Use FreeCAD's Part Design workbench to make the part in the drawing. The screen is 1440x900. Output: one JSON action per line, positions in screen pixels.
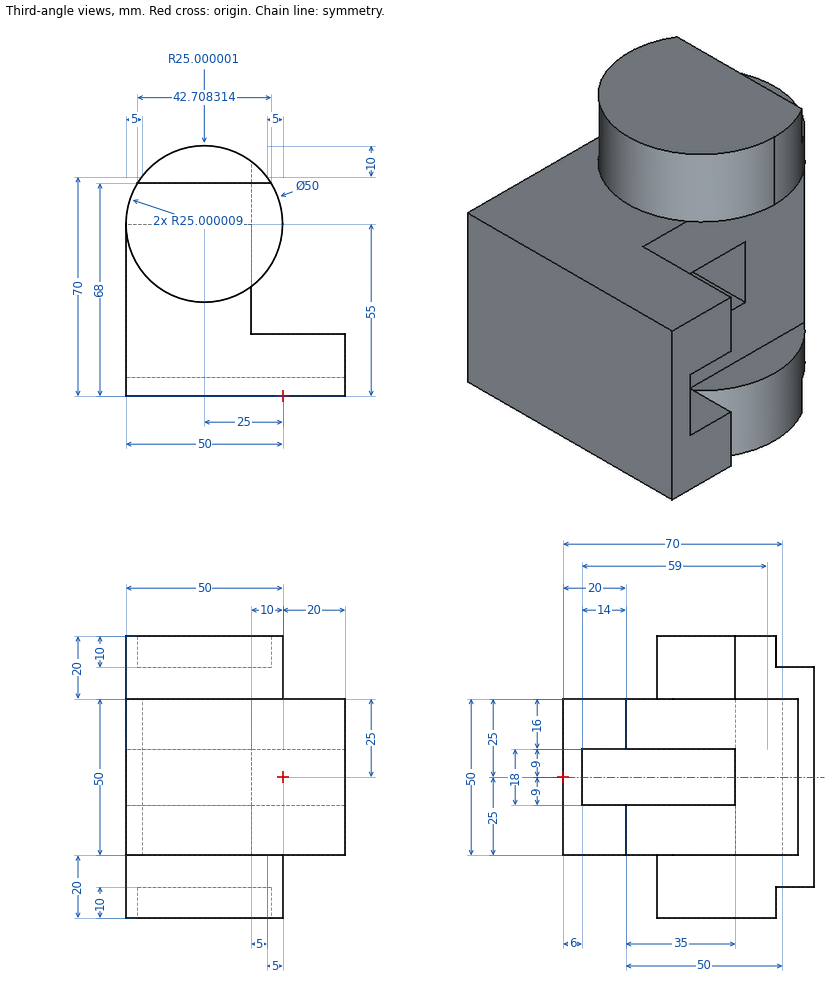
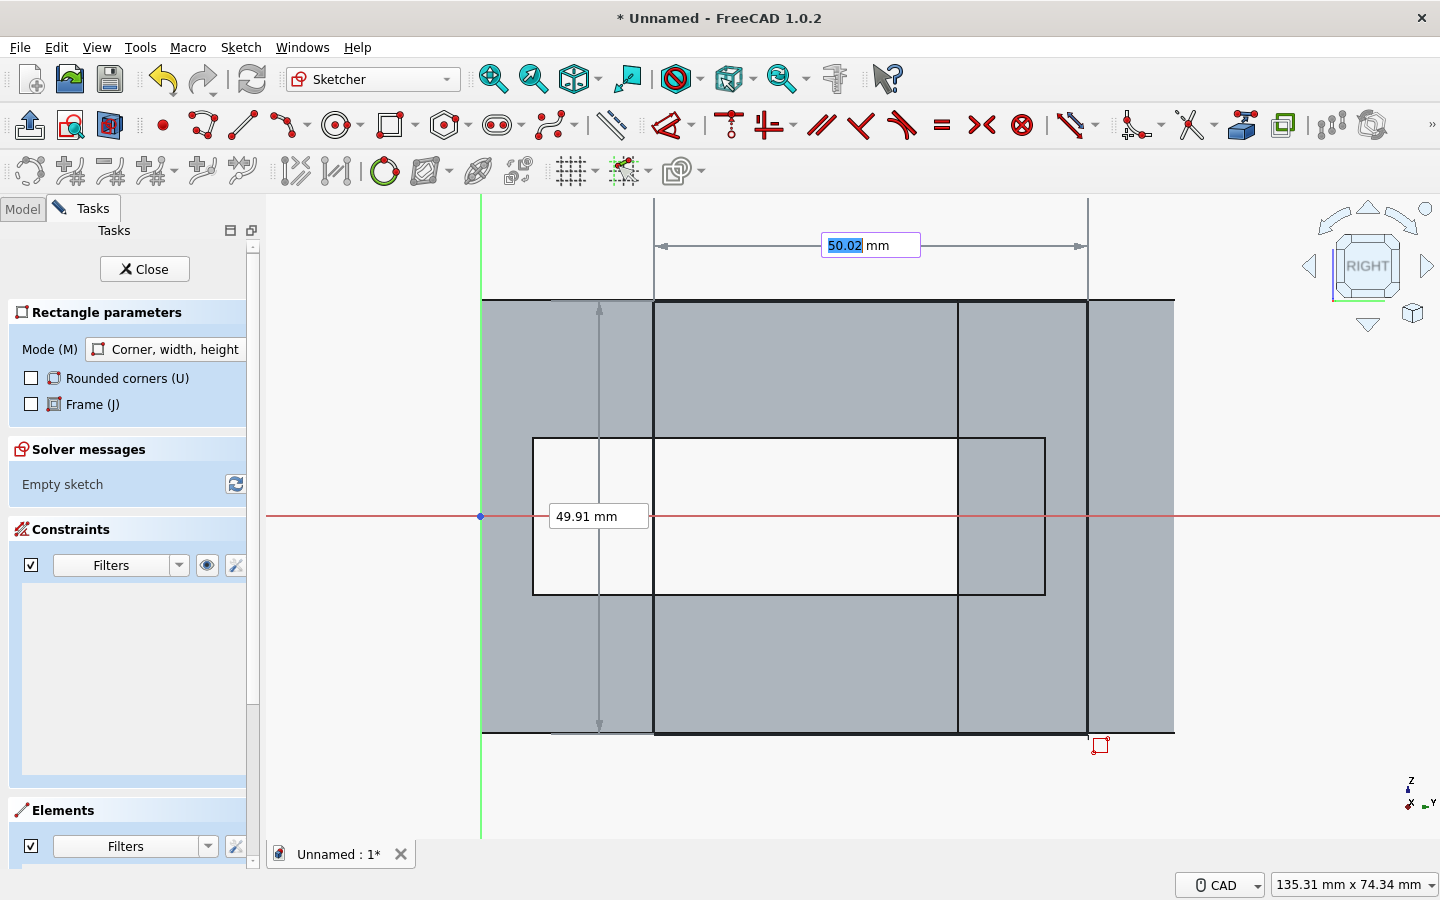
{"action": "type", "text": "50"}
{"action": "key", "text": "Tab"}
{"action": "type", "text": "50"}
{"action": "key", "text": "Return"}
{"action": "key", "text": "Escape"}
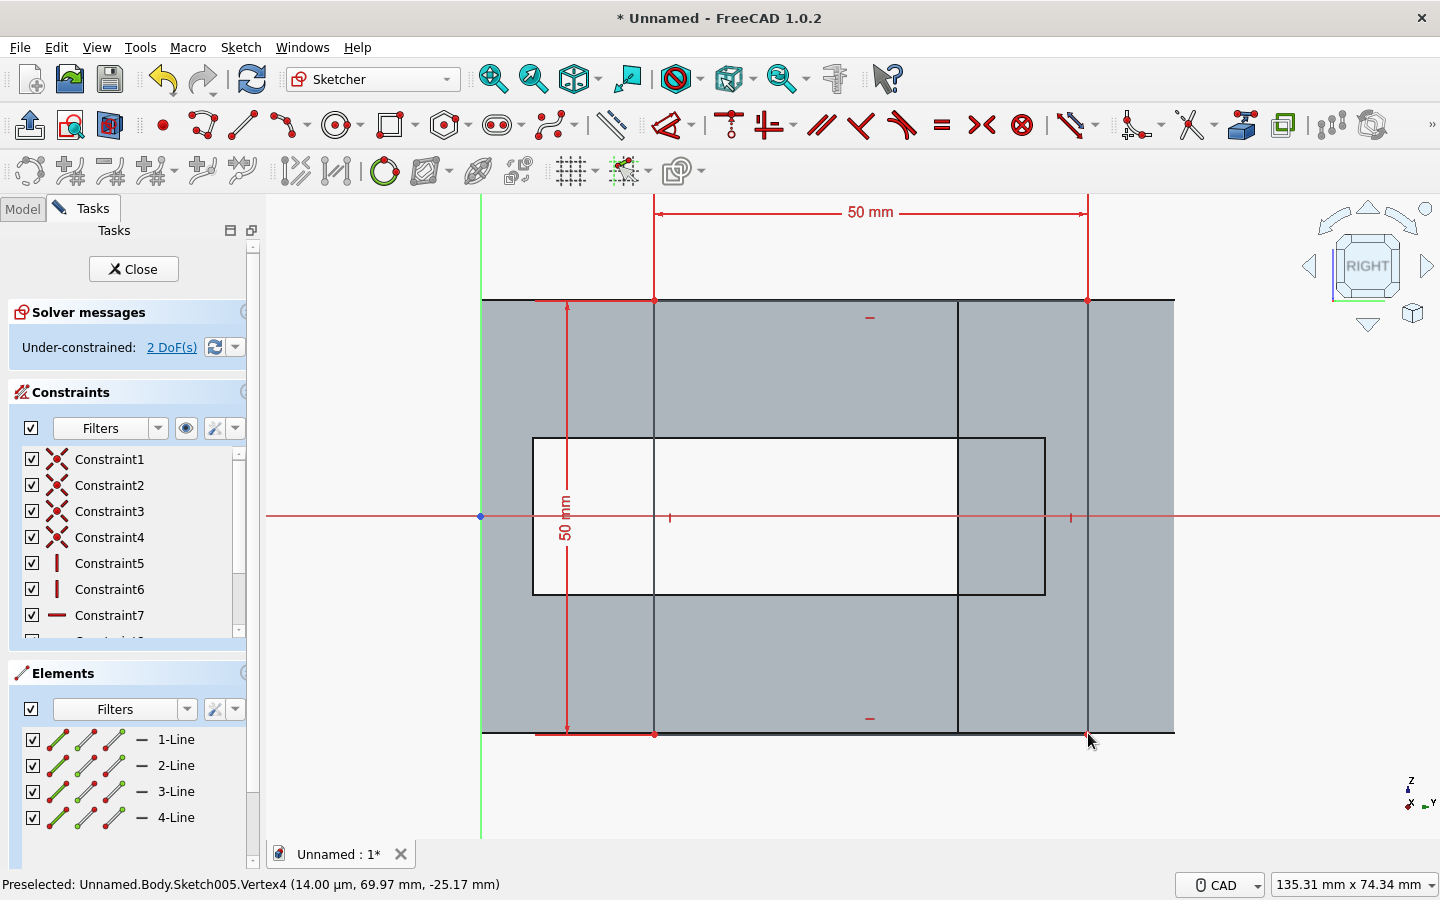
{"action": "key", "text": "d"}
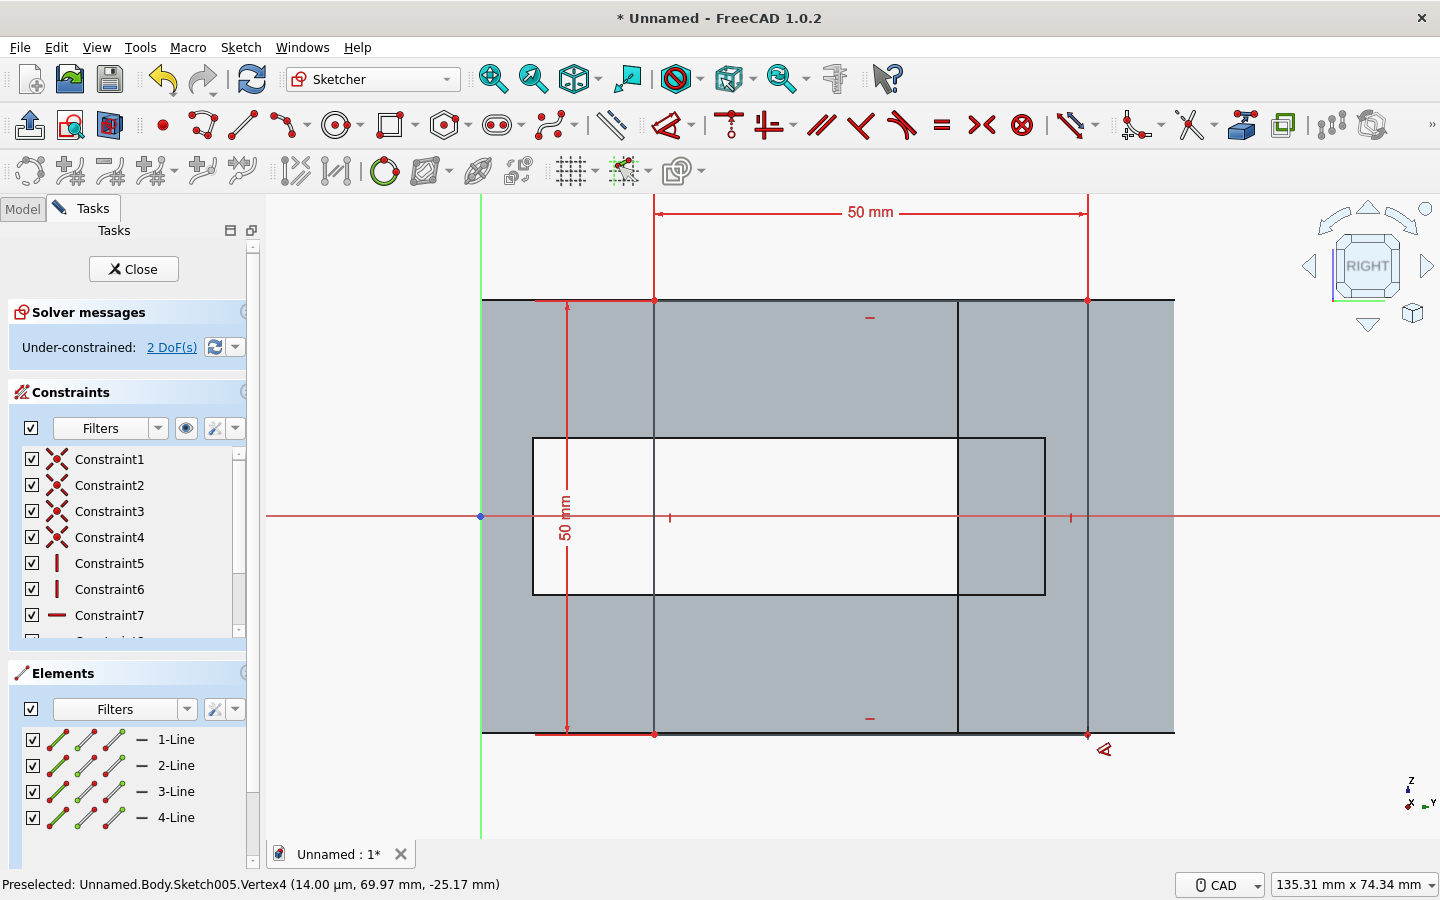
{"action": "left_click", "coordinate": [654, 301]}
{"action": "left_click", "coordinate": [567, 267]}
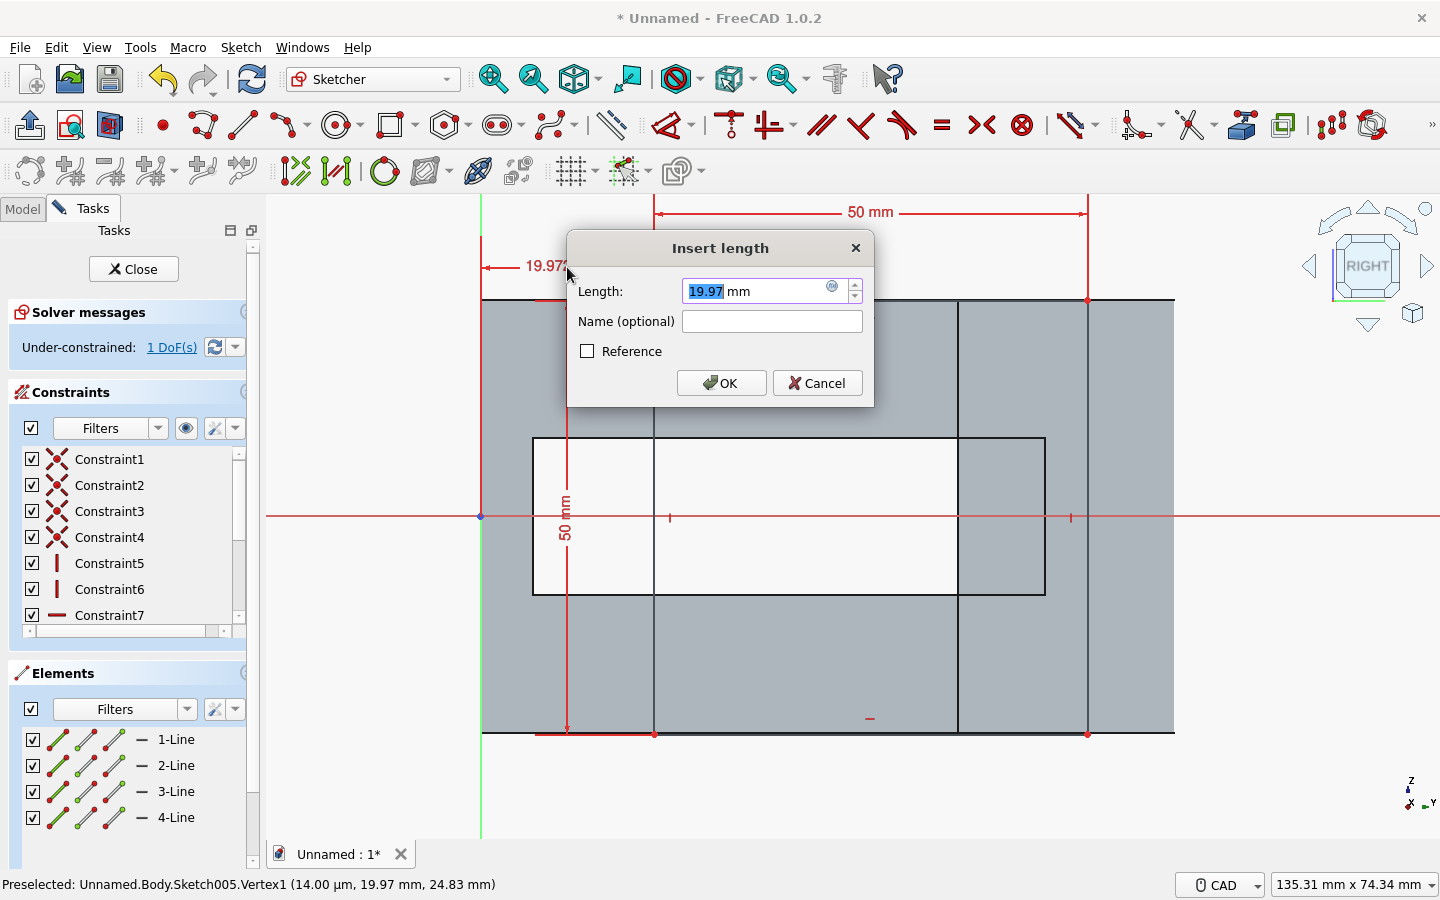
{"action": "type", "text": "20"}
{"action": "key", "text": "Return"}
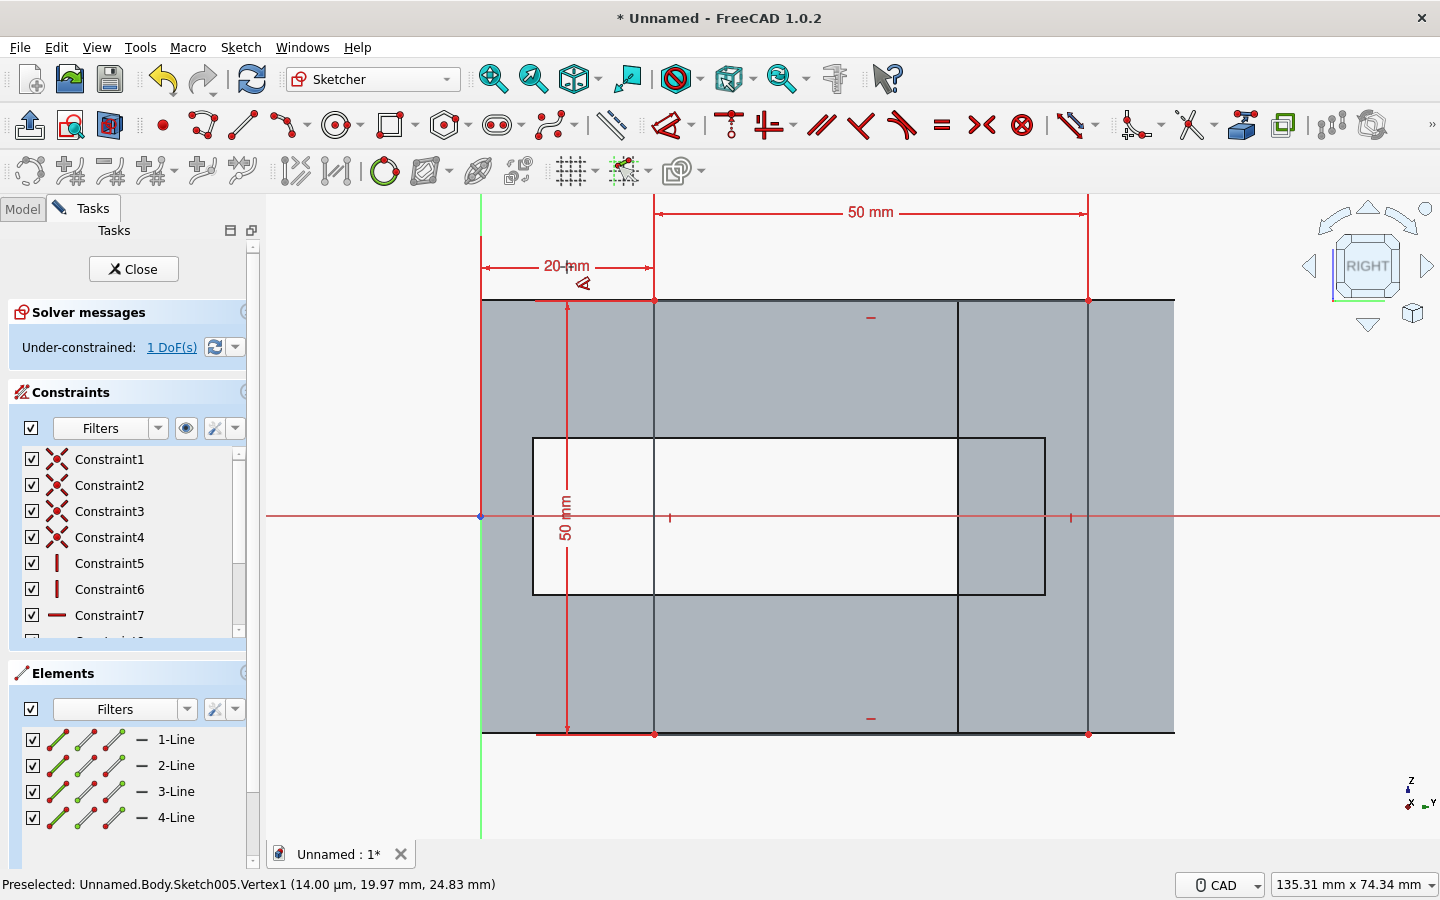
{"action": "left_click", "coordinate": [654, 301]}
{"action": "left_click", "coordinate": [447, 409]}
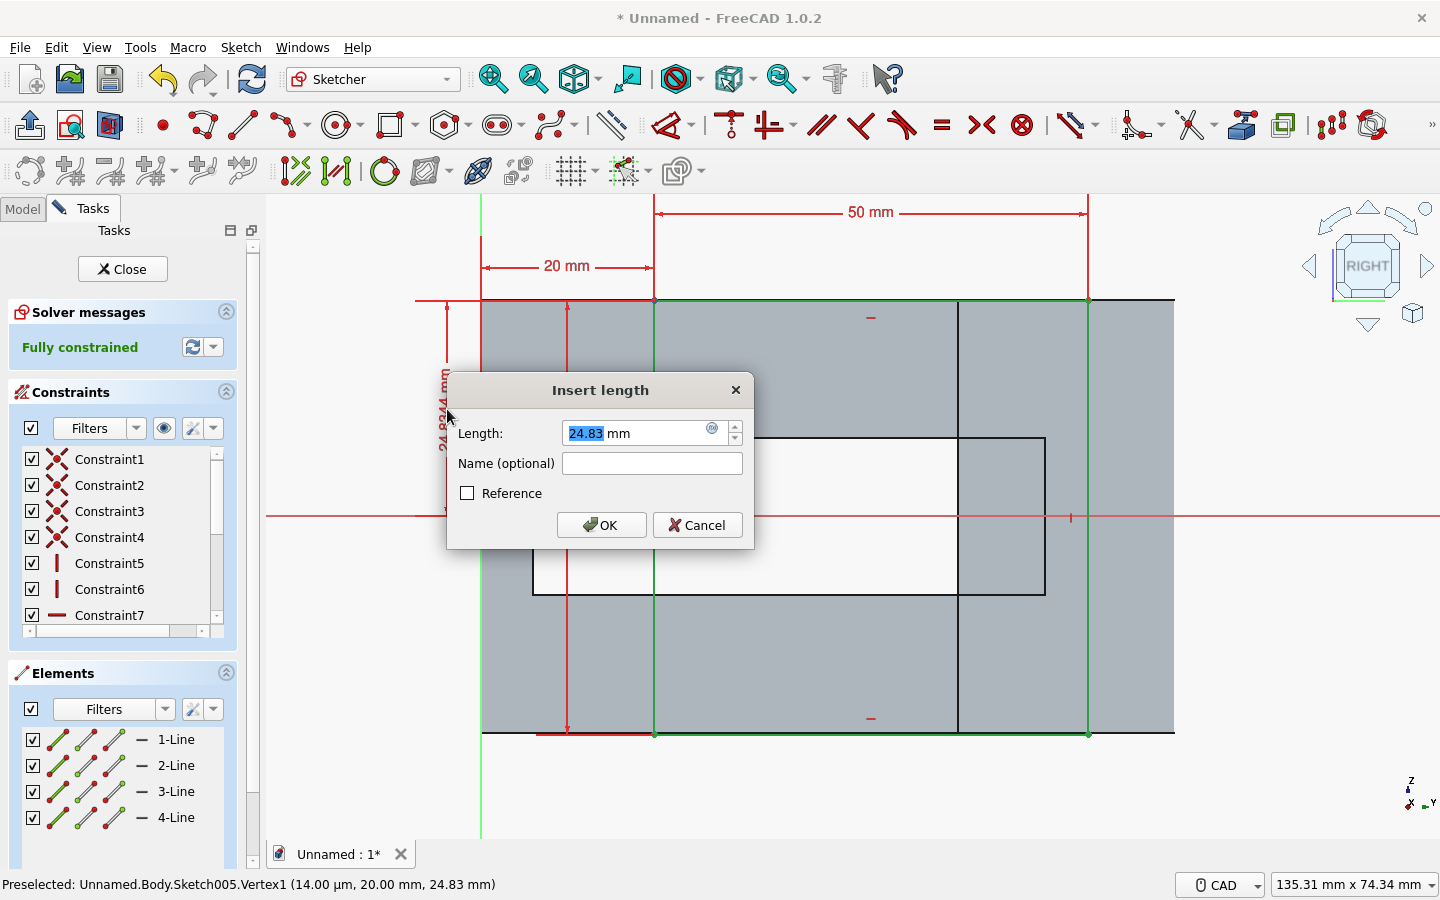
{"action": "type", "text": "25"}
{"action": "key", "text": "Return"}
{"action": "key", "text": "Escape"}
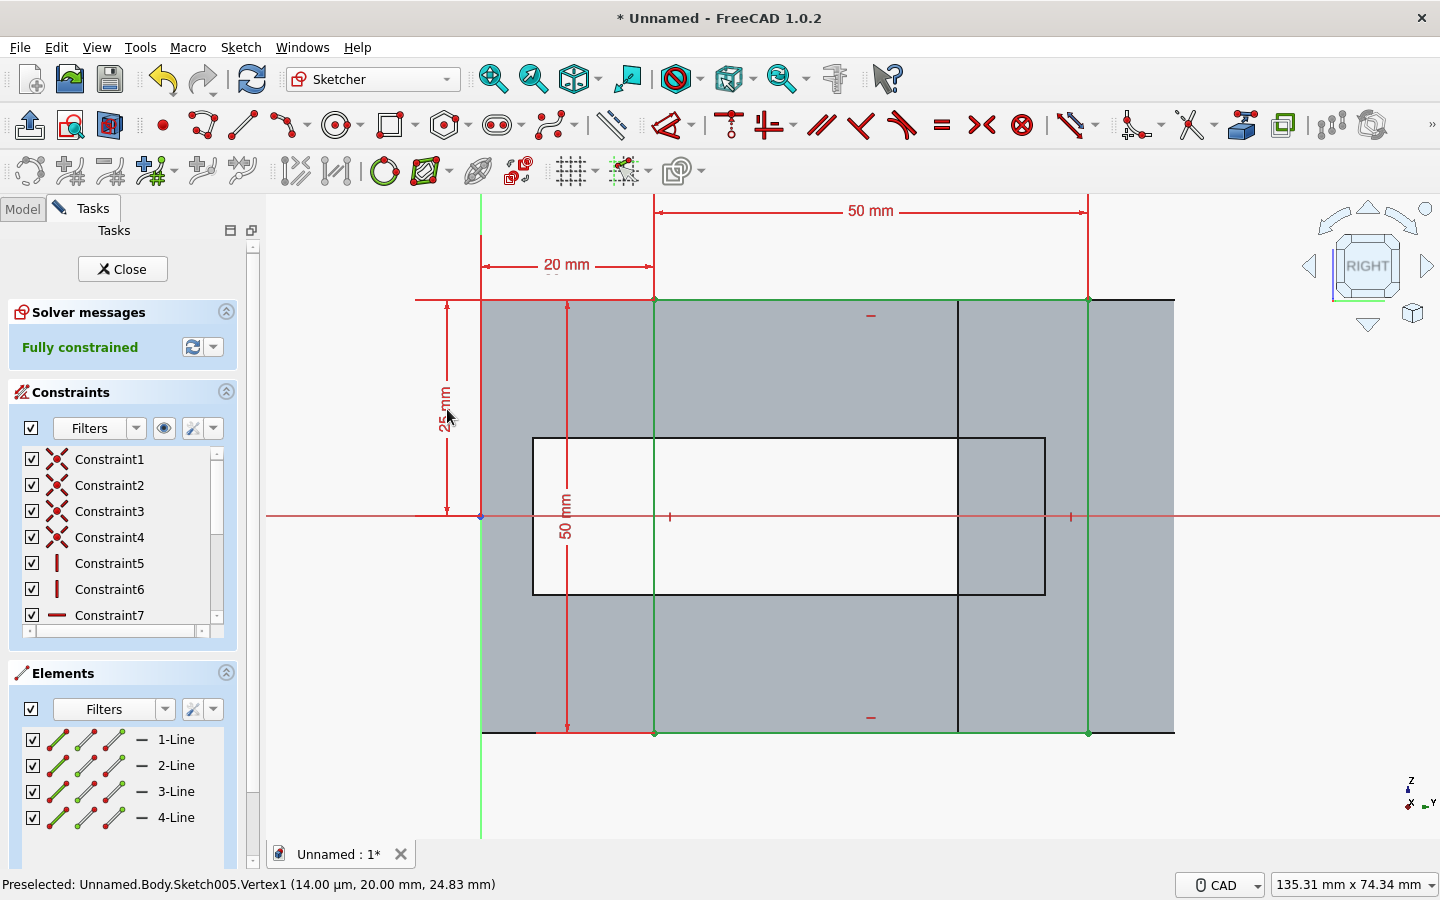
{"action": "left_click", "coordinate": [123, 269]}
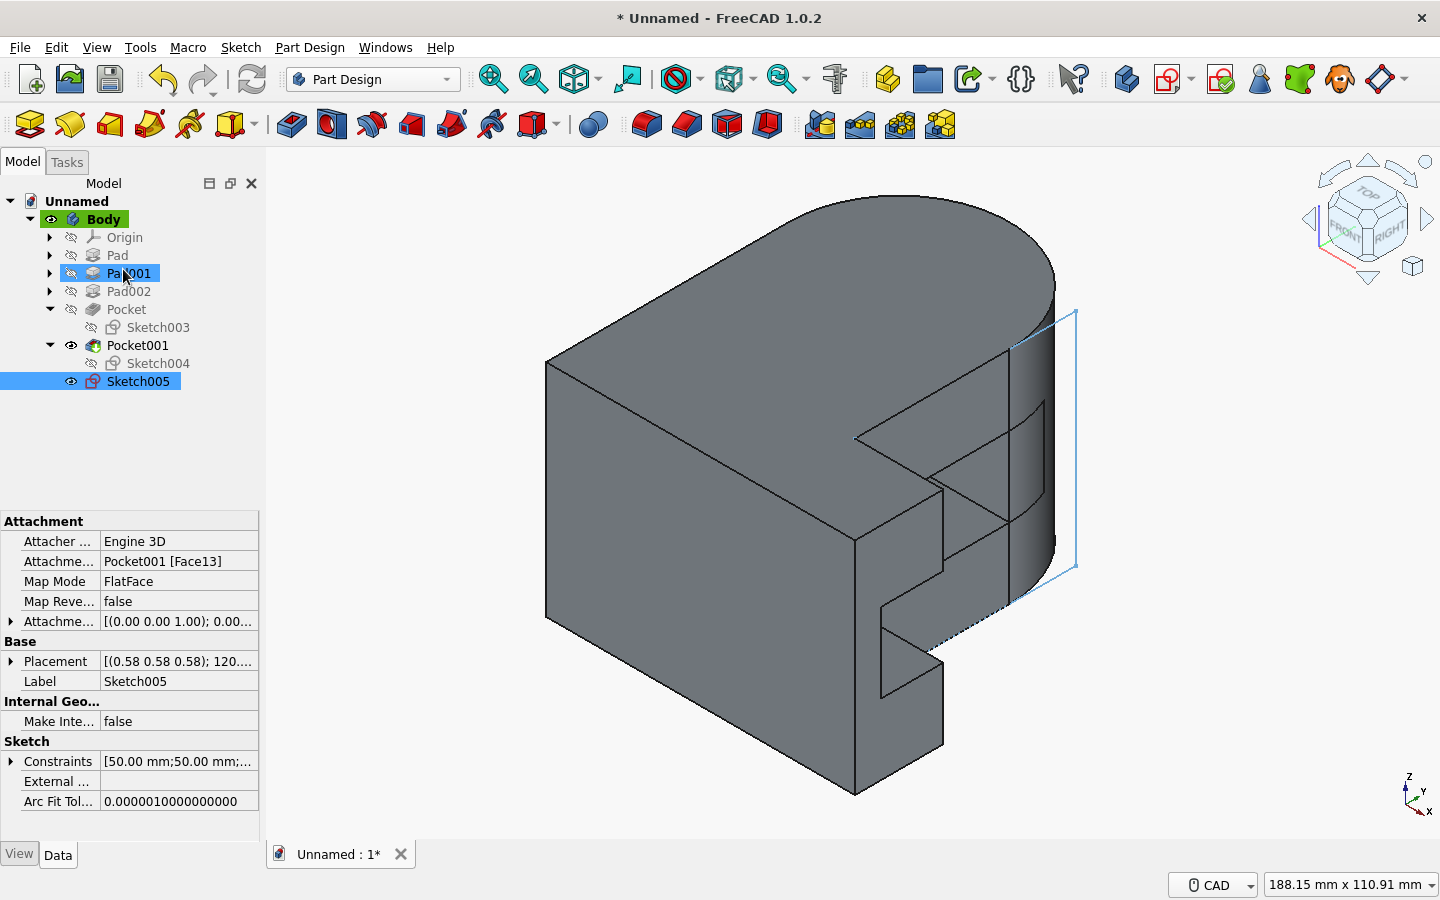
{"action": "left_click", "coordinate": [292, 124]}